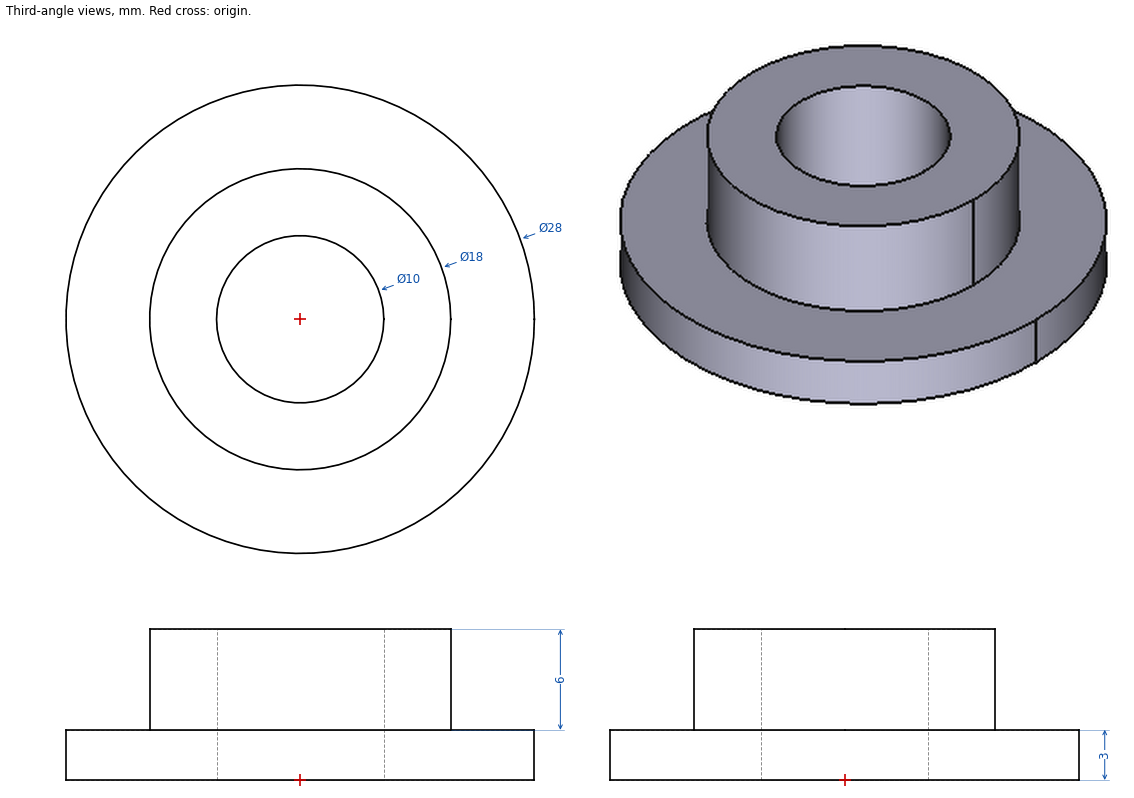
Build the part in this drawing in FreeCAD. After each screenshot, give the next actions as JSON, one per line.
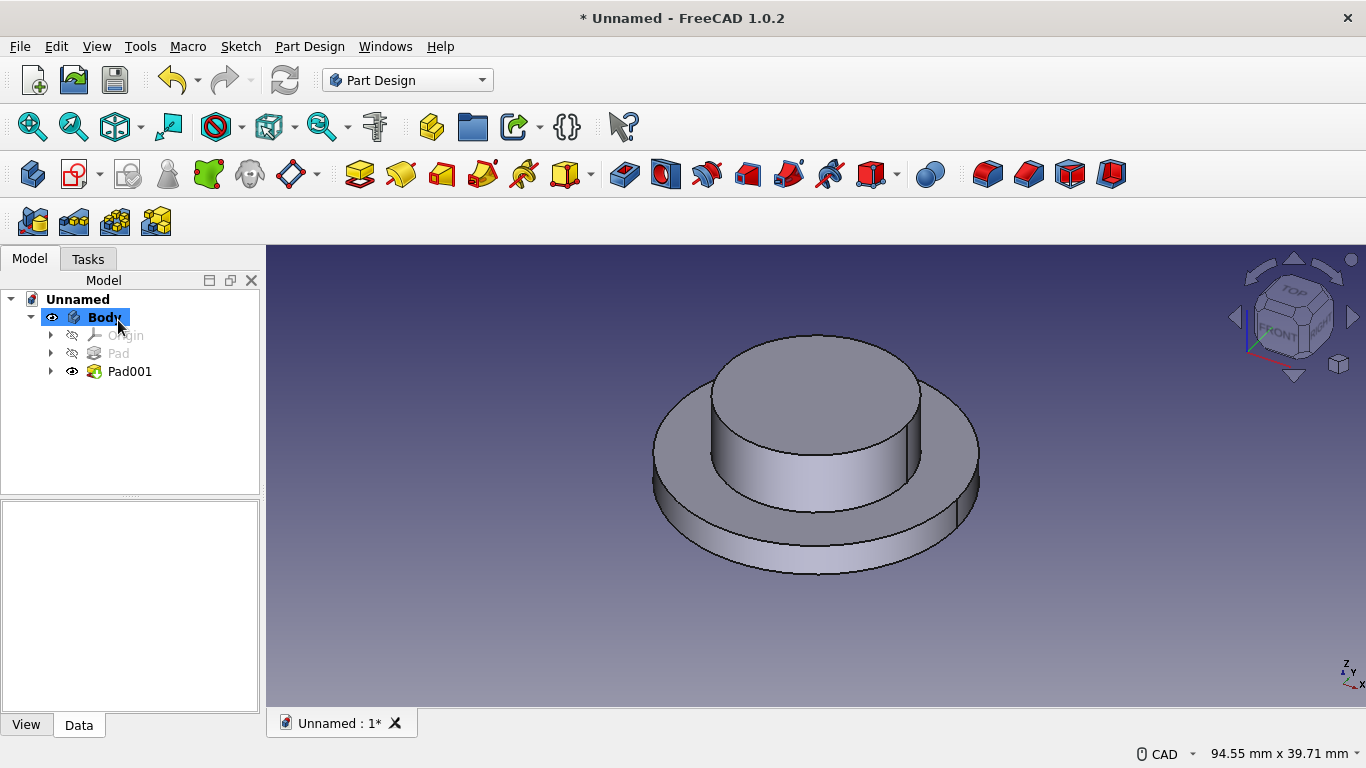
{"action": "left_click", "coordinate": [816, 394]}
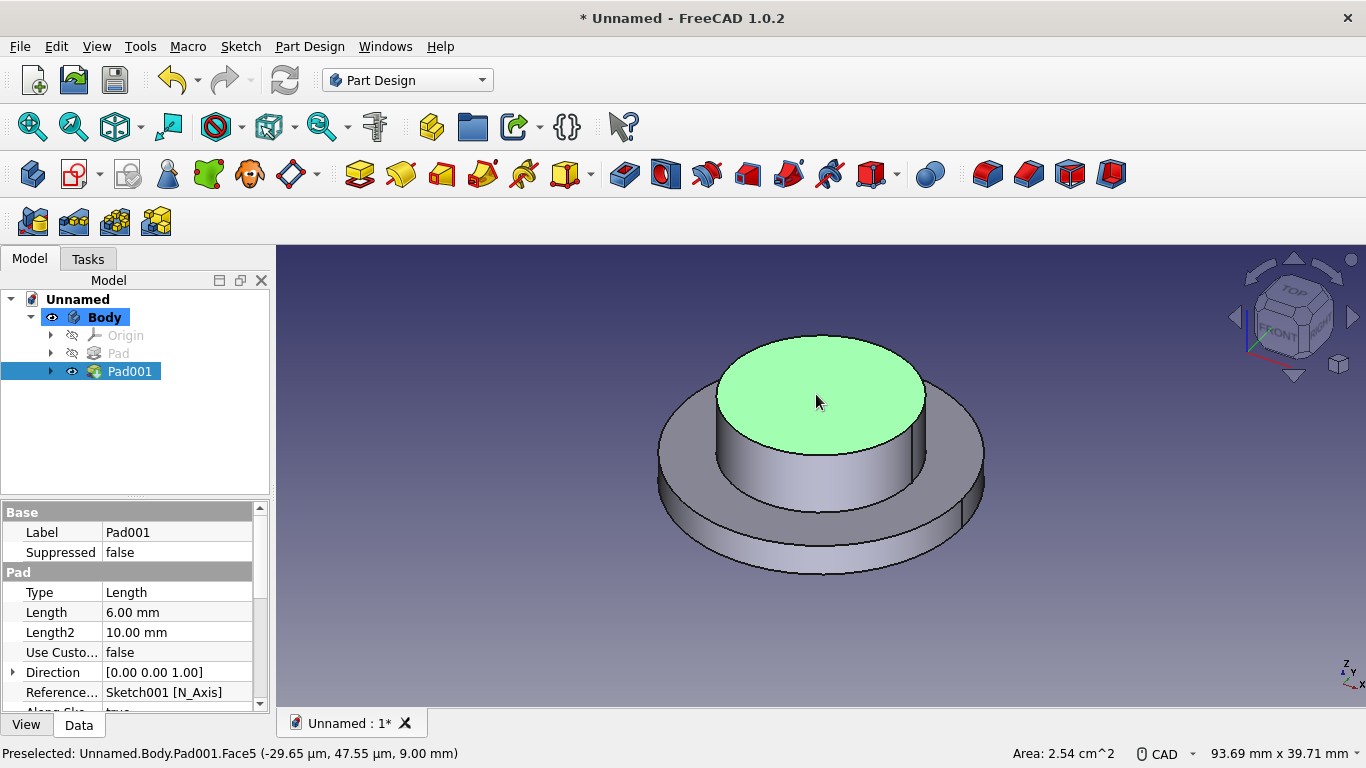
{"action": "left_click", "coordinate": [74, 174]}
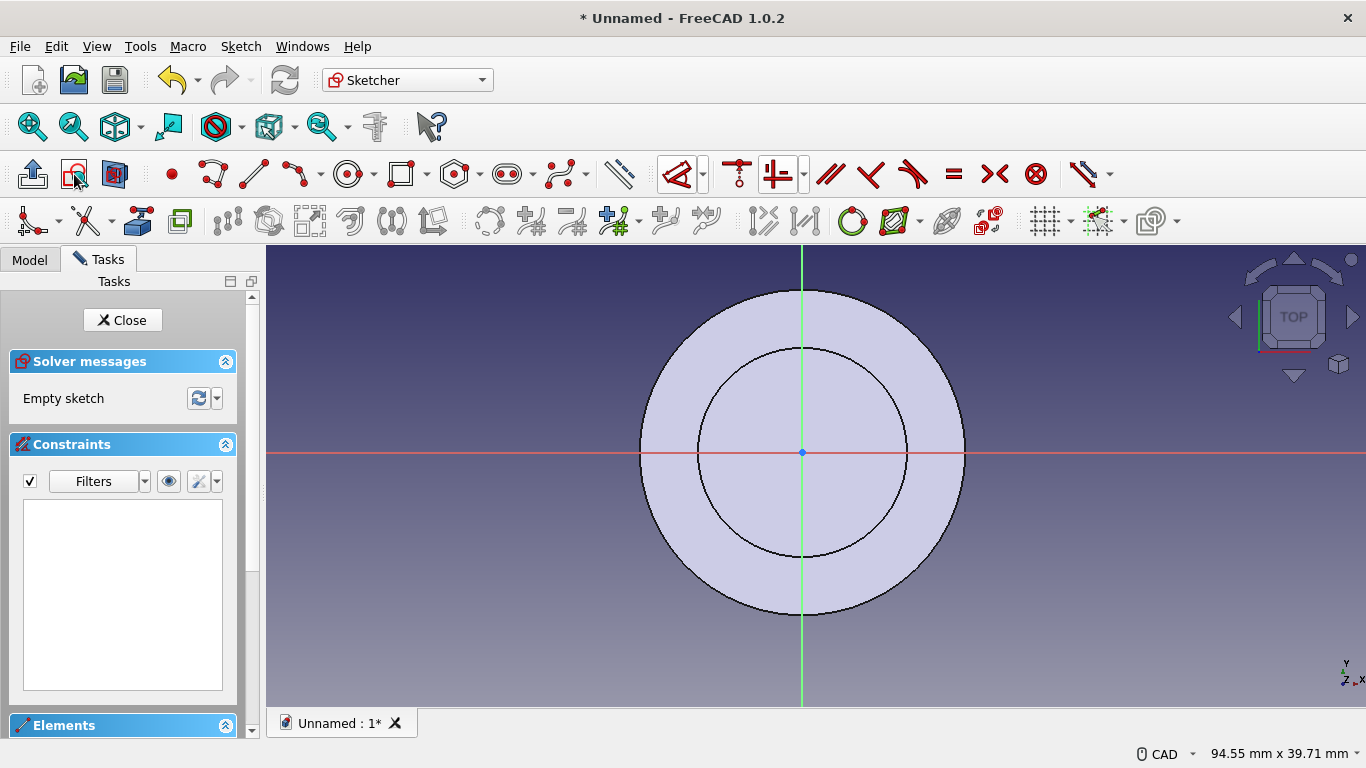
{"action": "scroll", "coordinate": [834, 439], "scroll_direction": "up", "scroll_amount": 5}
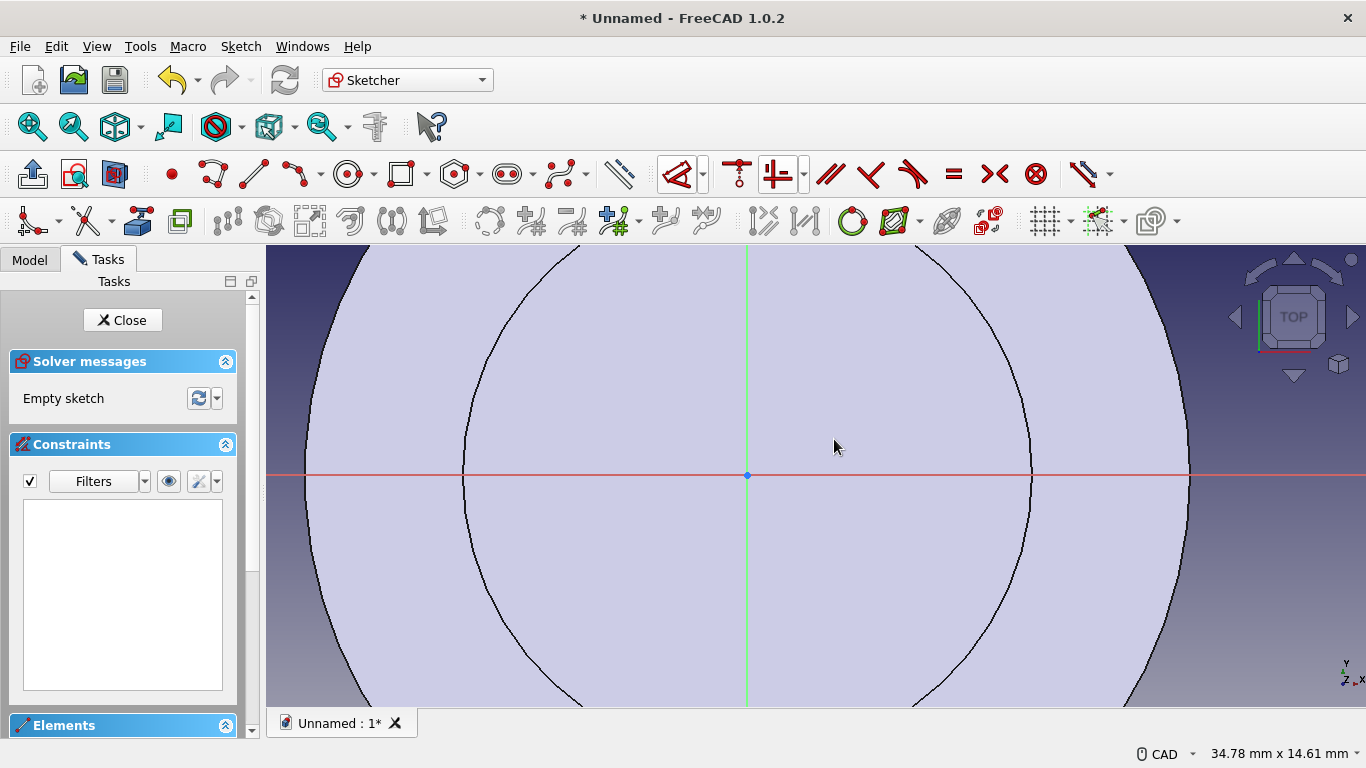
{"action": "key", "text": "g c"}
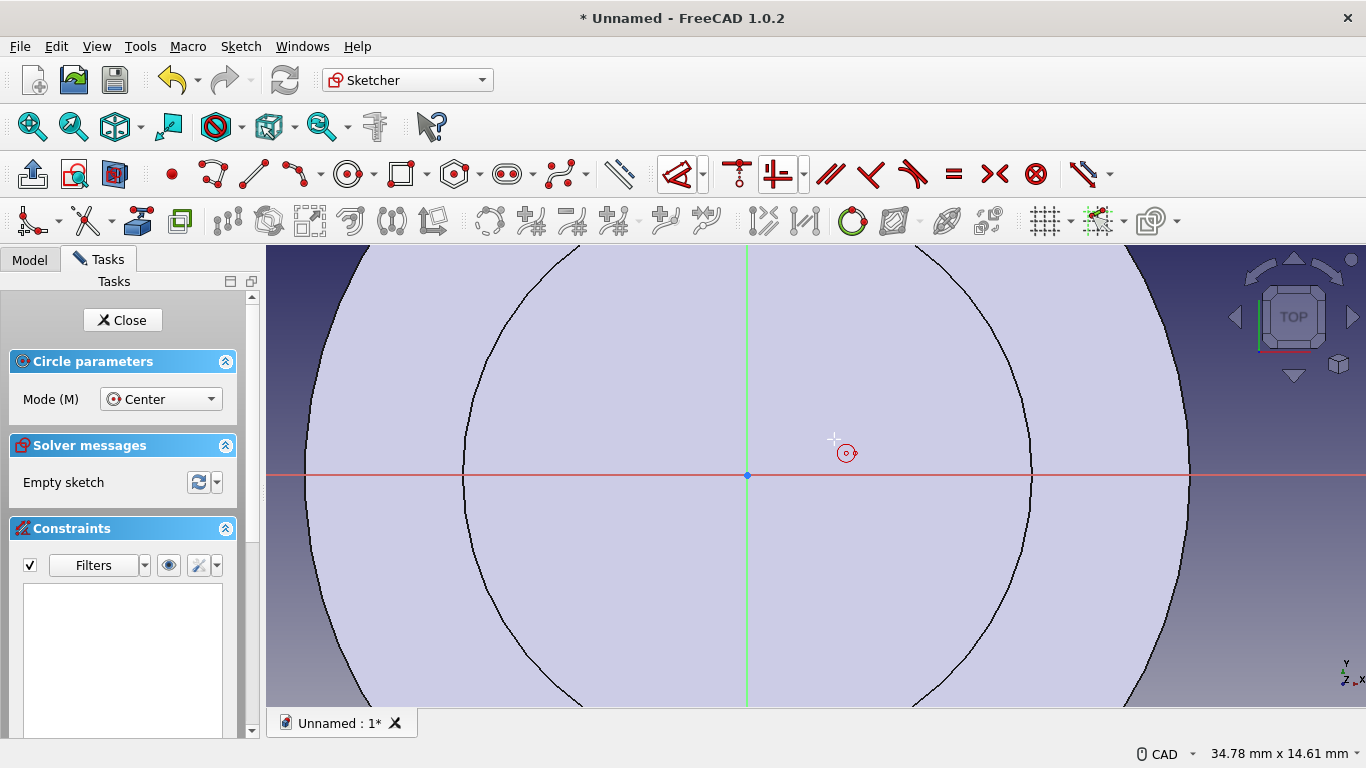
{"action": "left_click", "coordinate": [747, 475]}
{"action": "left_click", "coordinate": [859, 363]}
{"action": "key", "text": "Escape"}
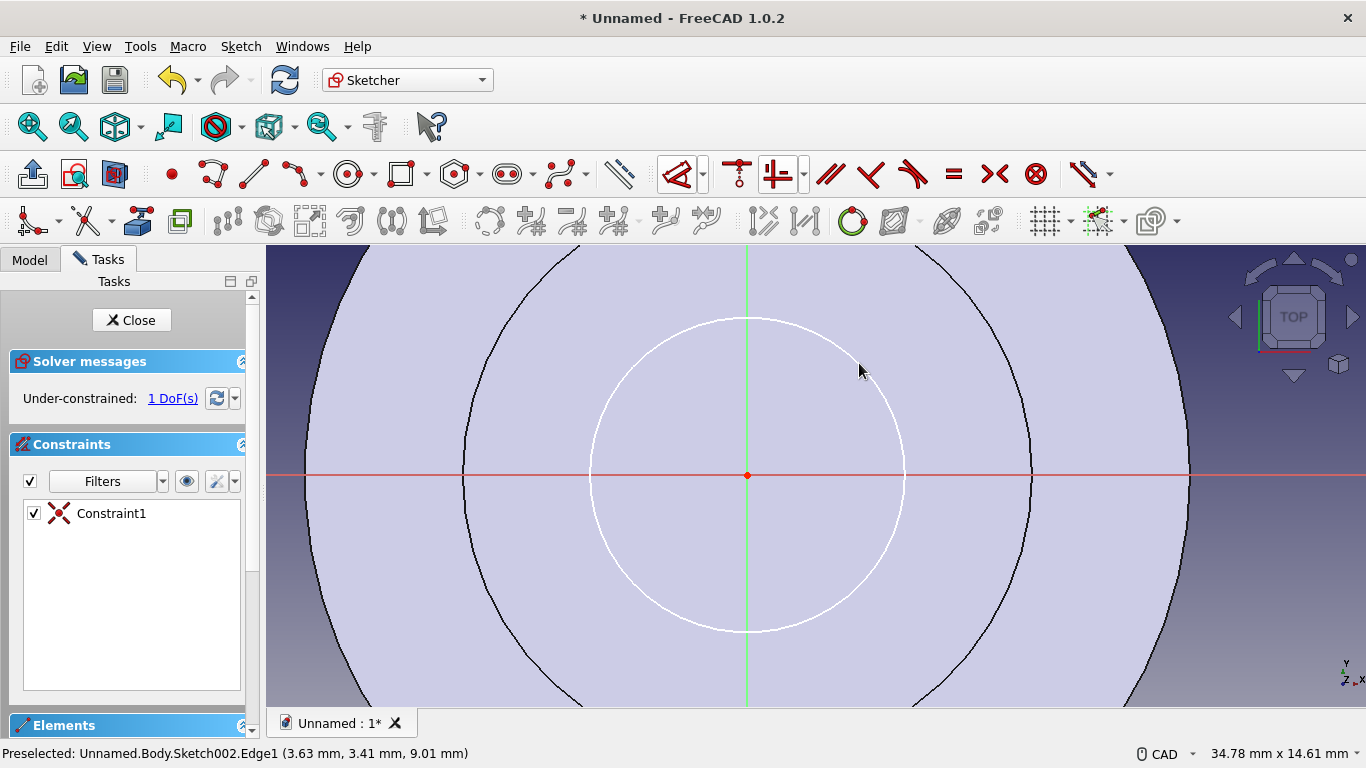
{"action": "left_click", "coordinate": [858, 363]}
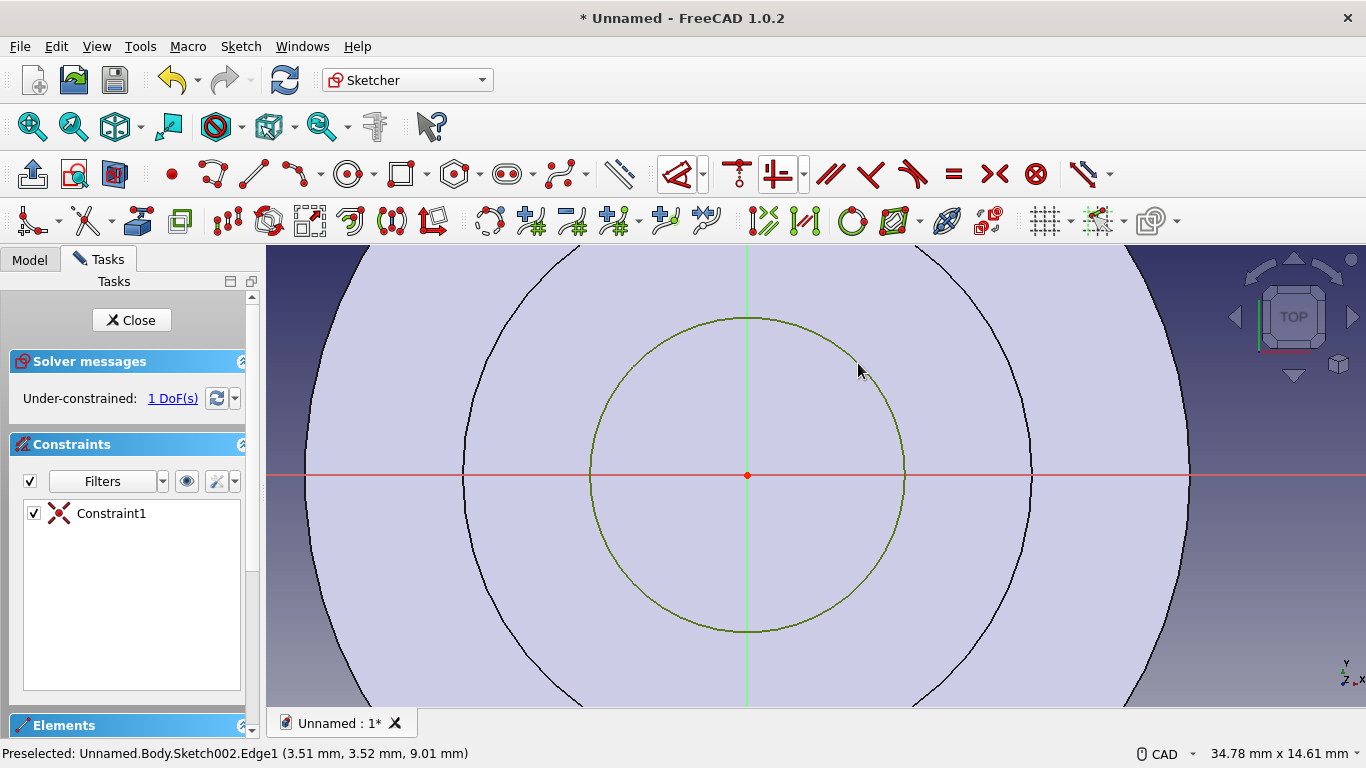
{"action": "key", "text": "k o"}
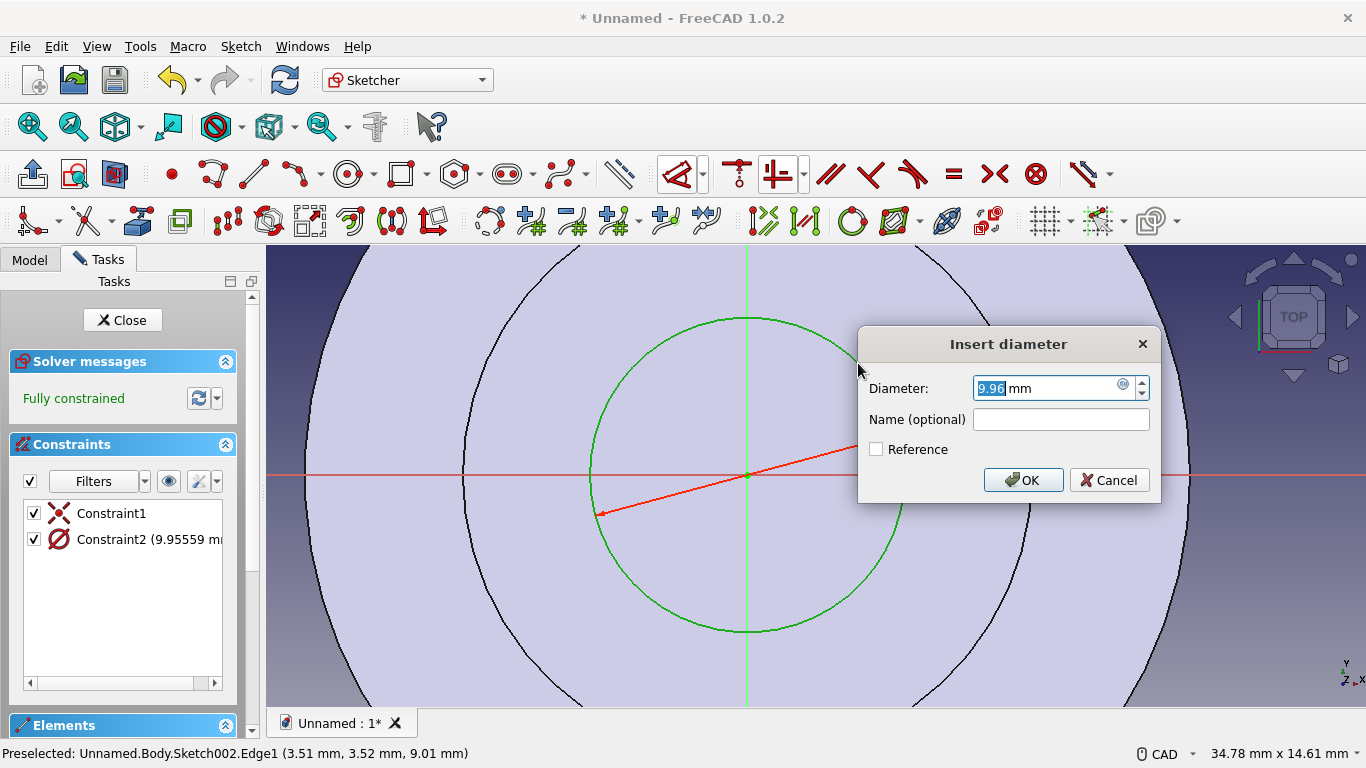
{"action": "type", "text": "10"}
{"action": "key", "text": "Return"}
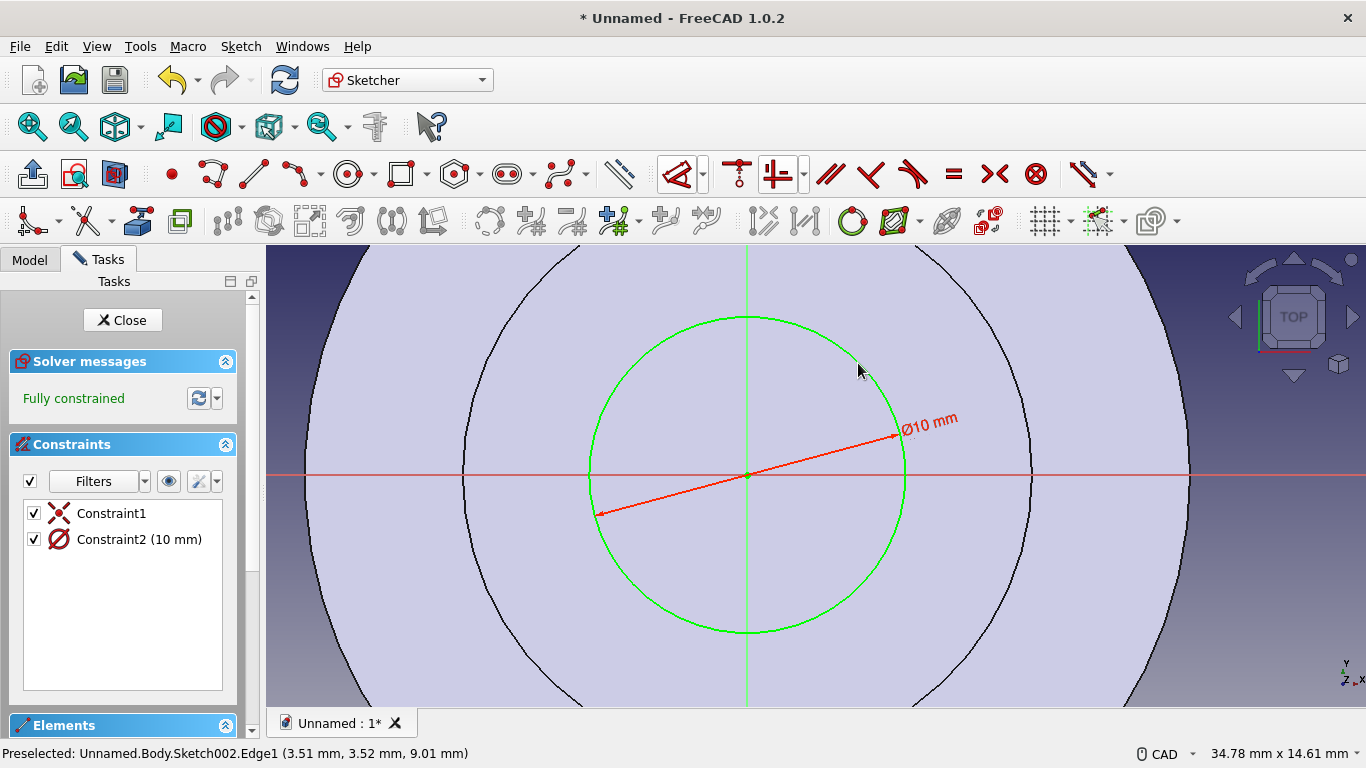
{"action": "left_click", "coordinate": [123, 320]}